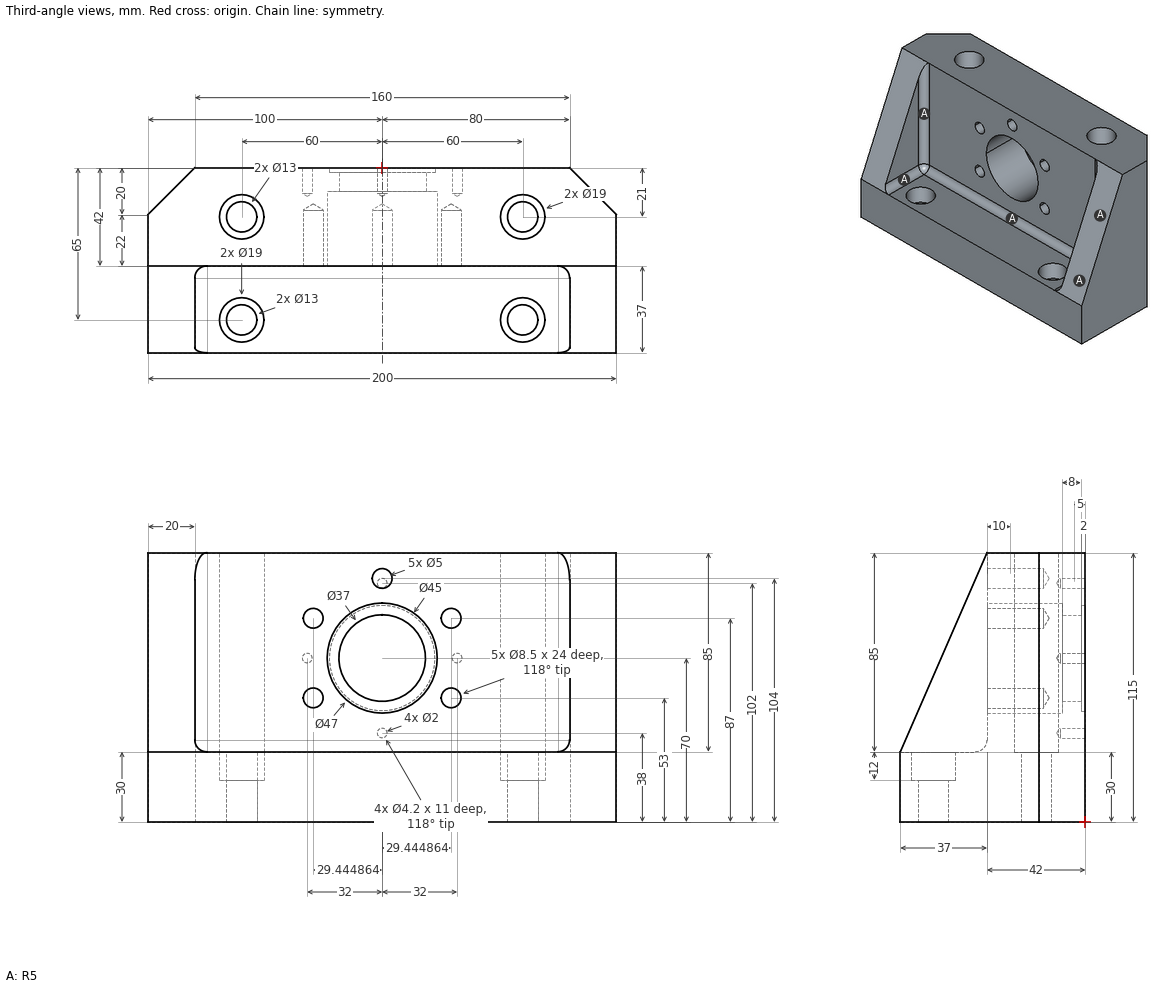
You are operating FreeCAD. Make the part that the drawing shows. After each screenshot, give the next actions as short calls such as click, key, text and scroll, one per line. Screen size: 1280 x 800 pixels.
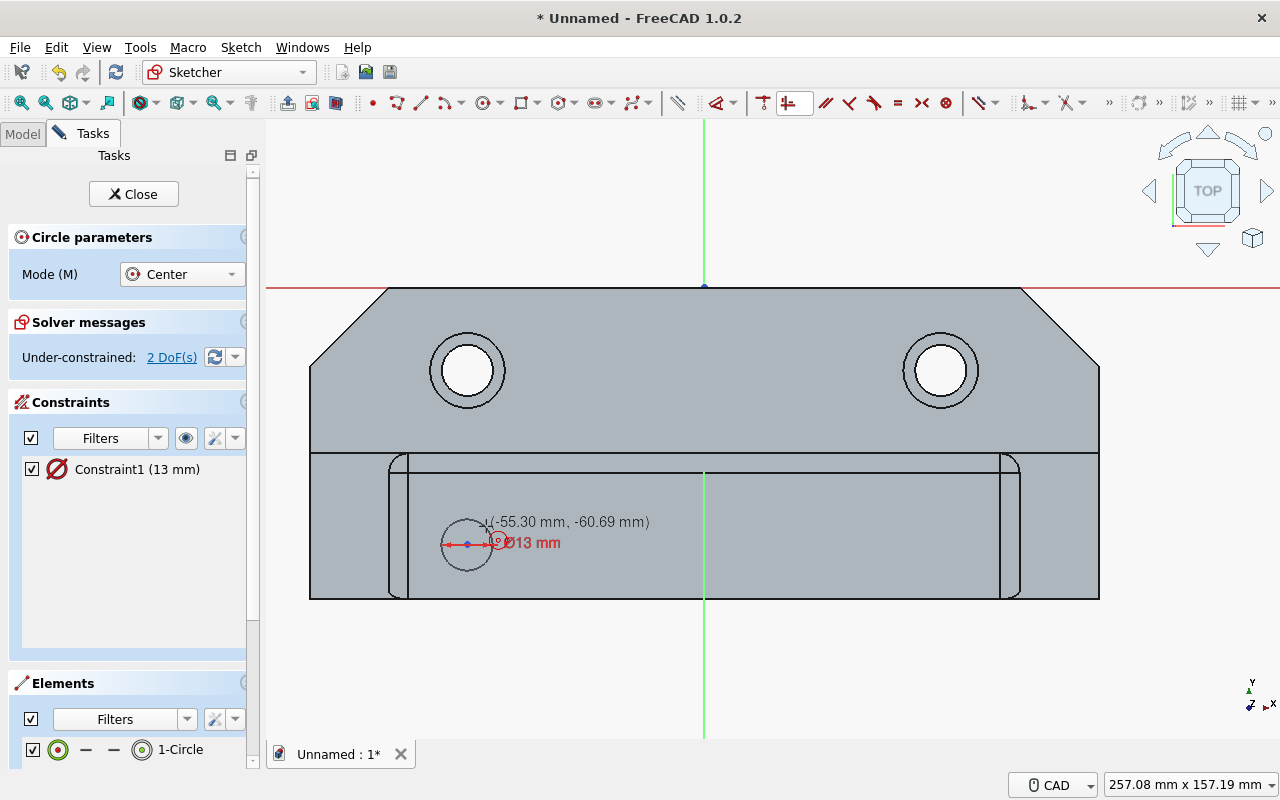
click(941, 544)
move(959, 526)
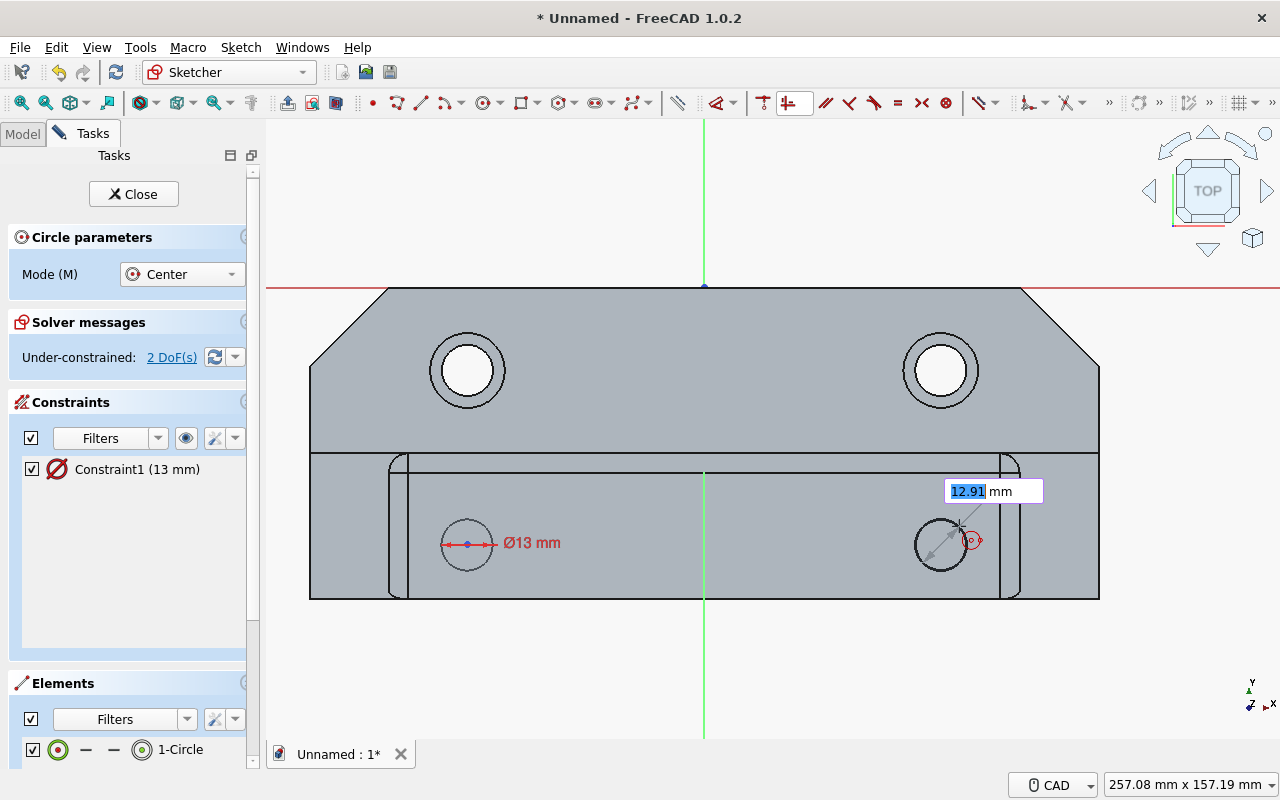
text(13)
key(Return)
key(Escape)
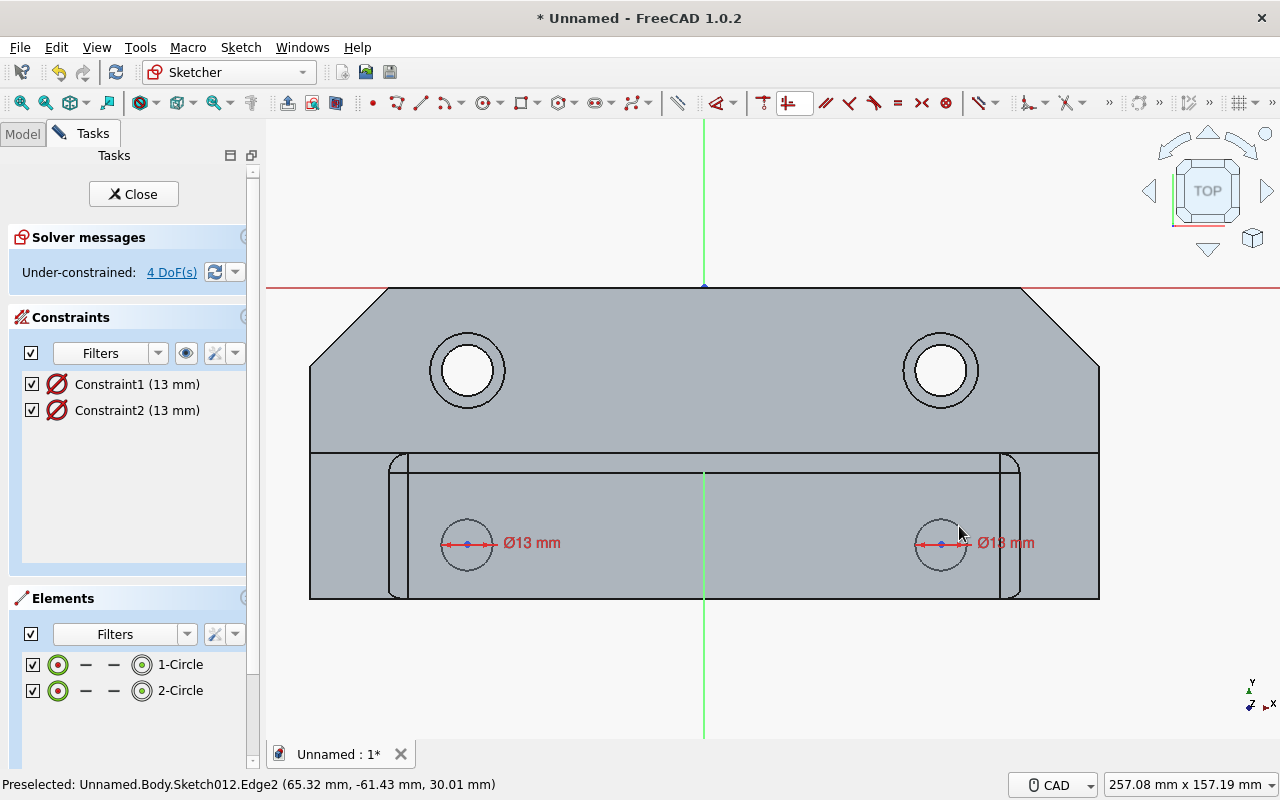
click(467, 545)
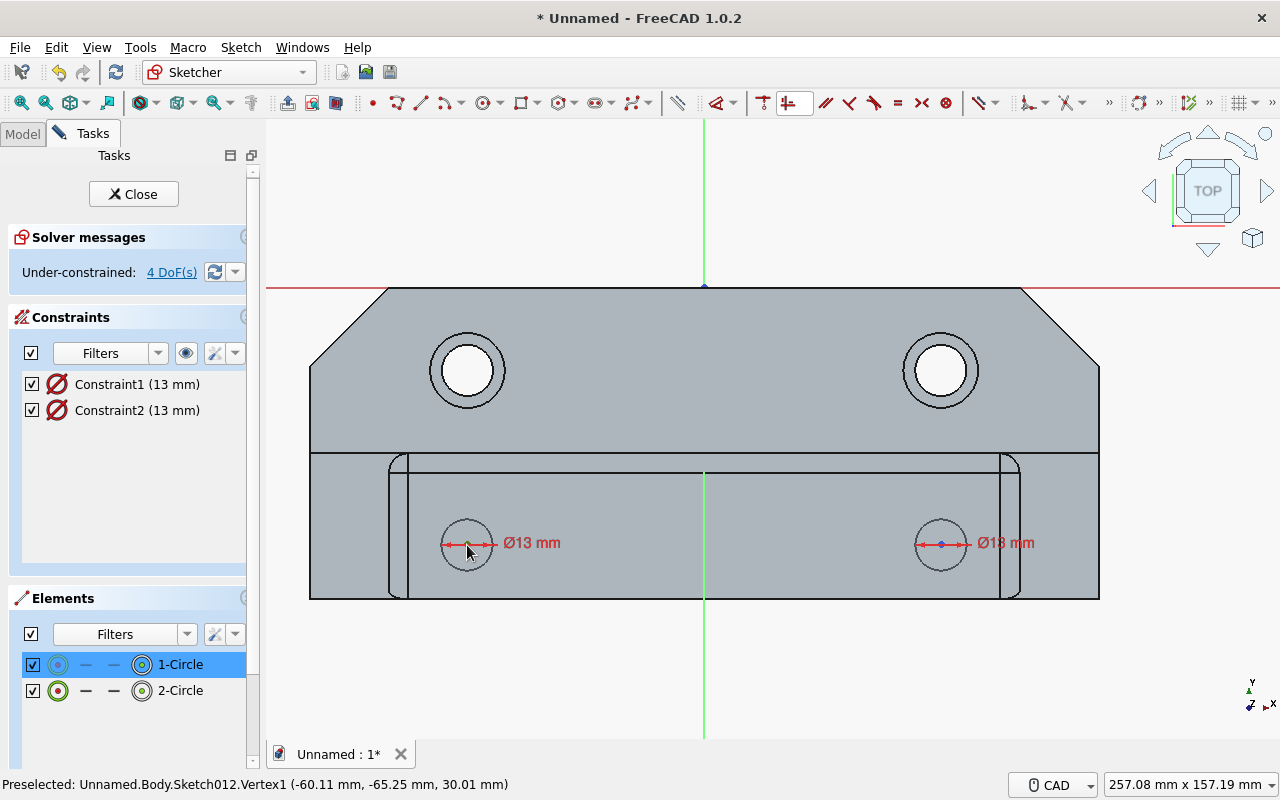
click(941, 545)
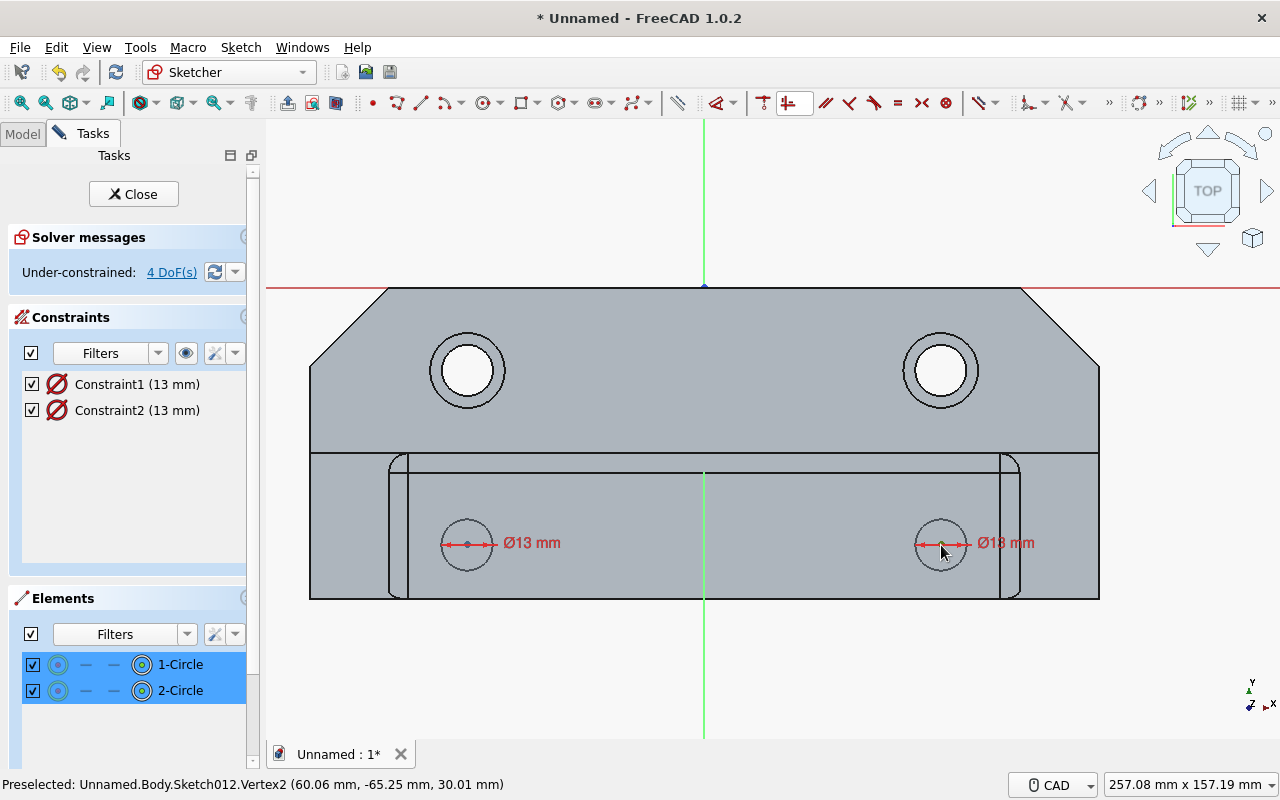
key(h)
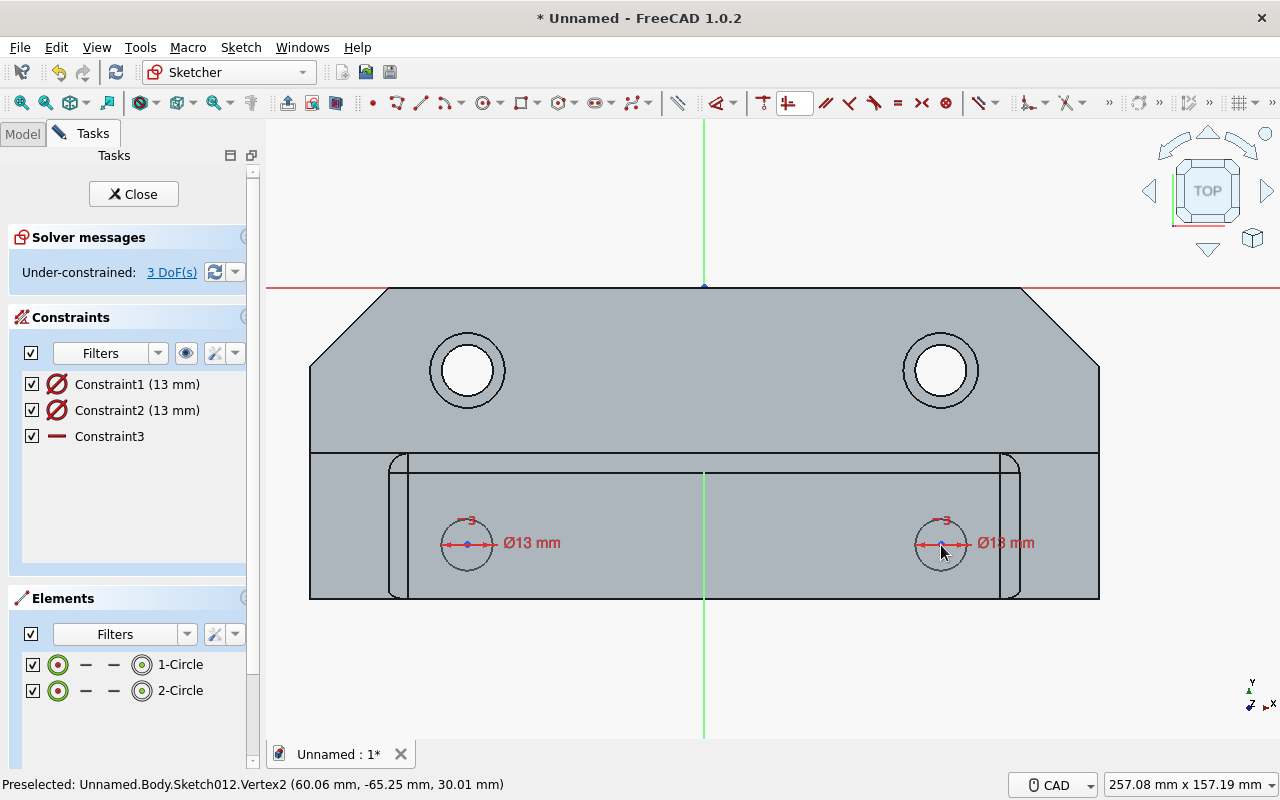
click(716, 104)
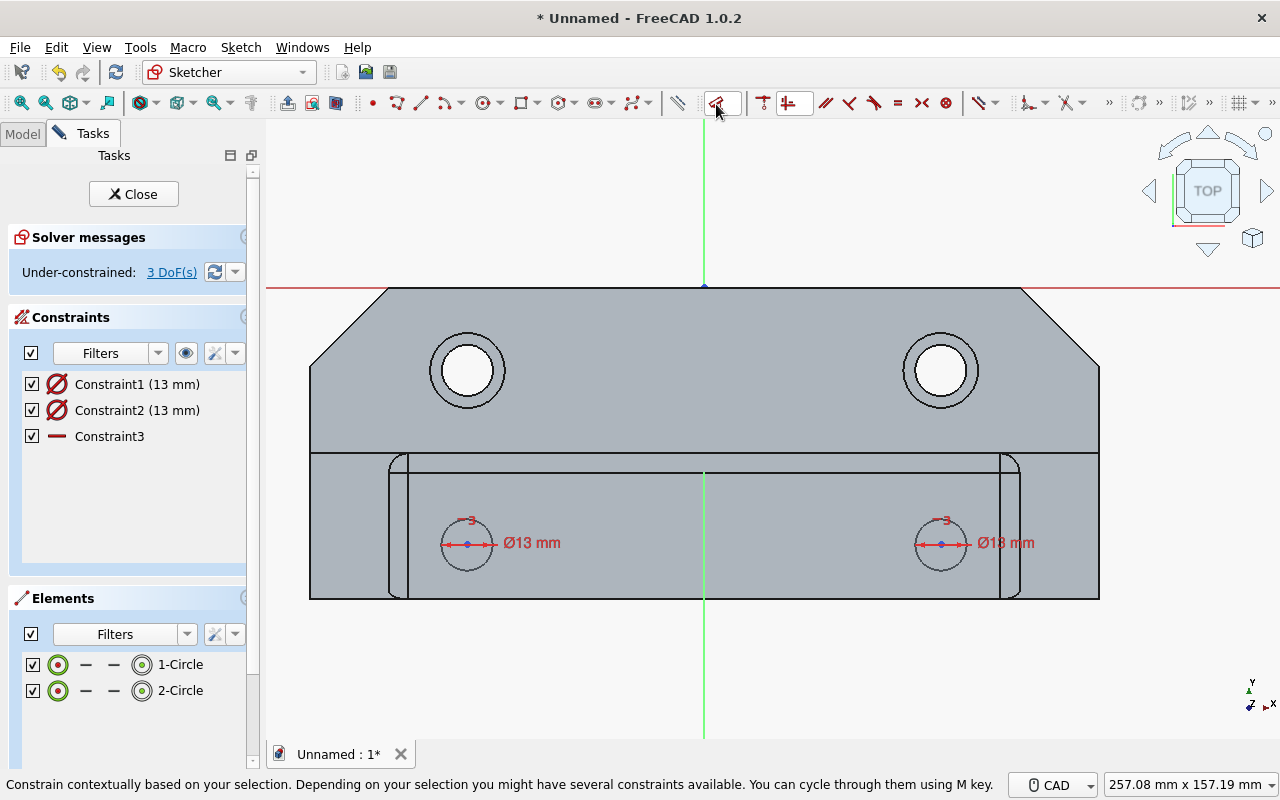
click(467, 545)
click(586, 254)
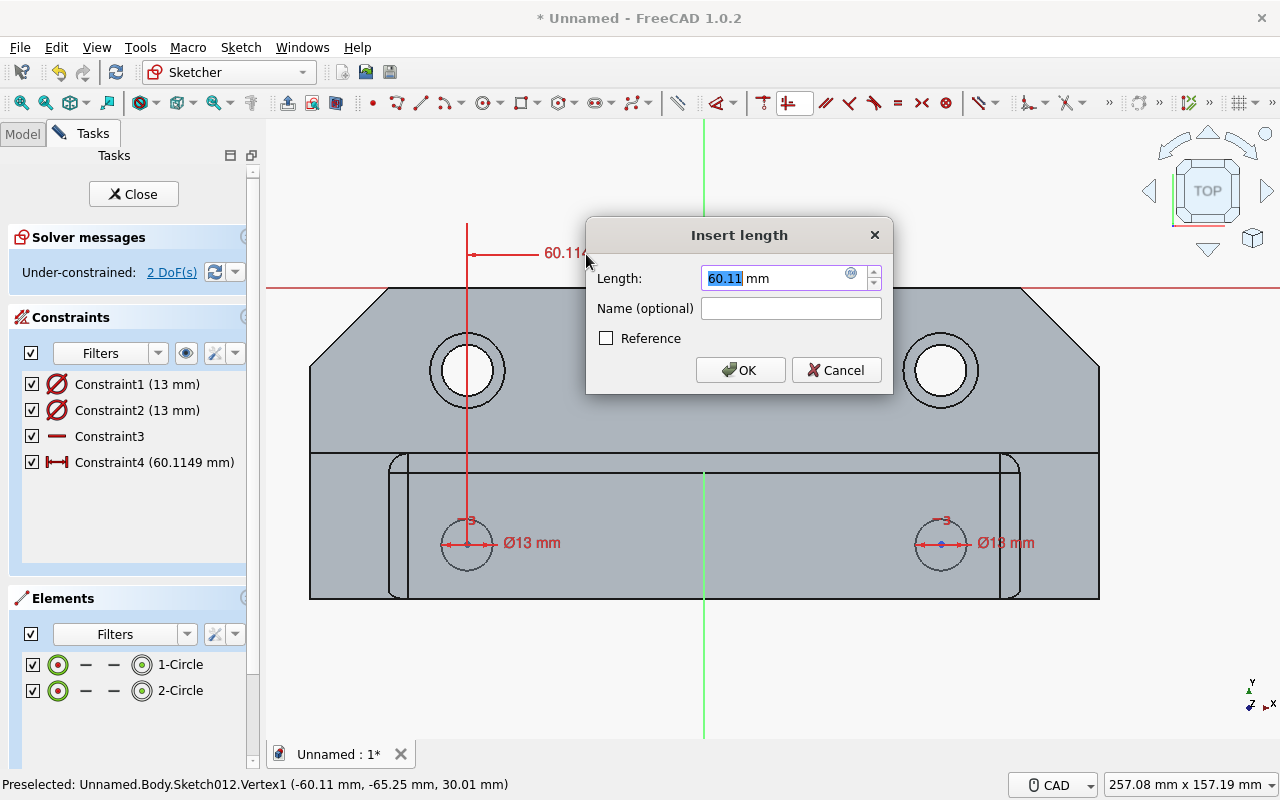
text(60)
key(Return)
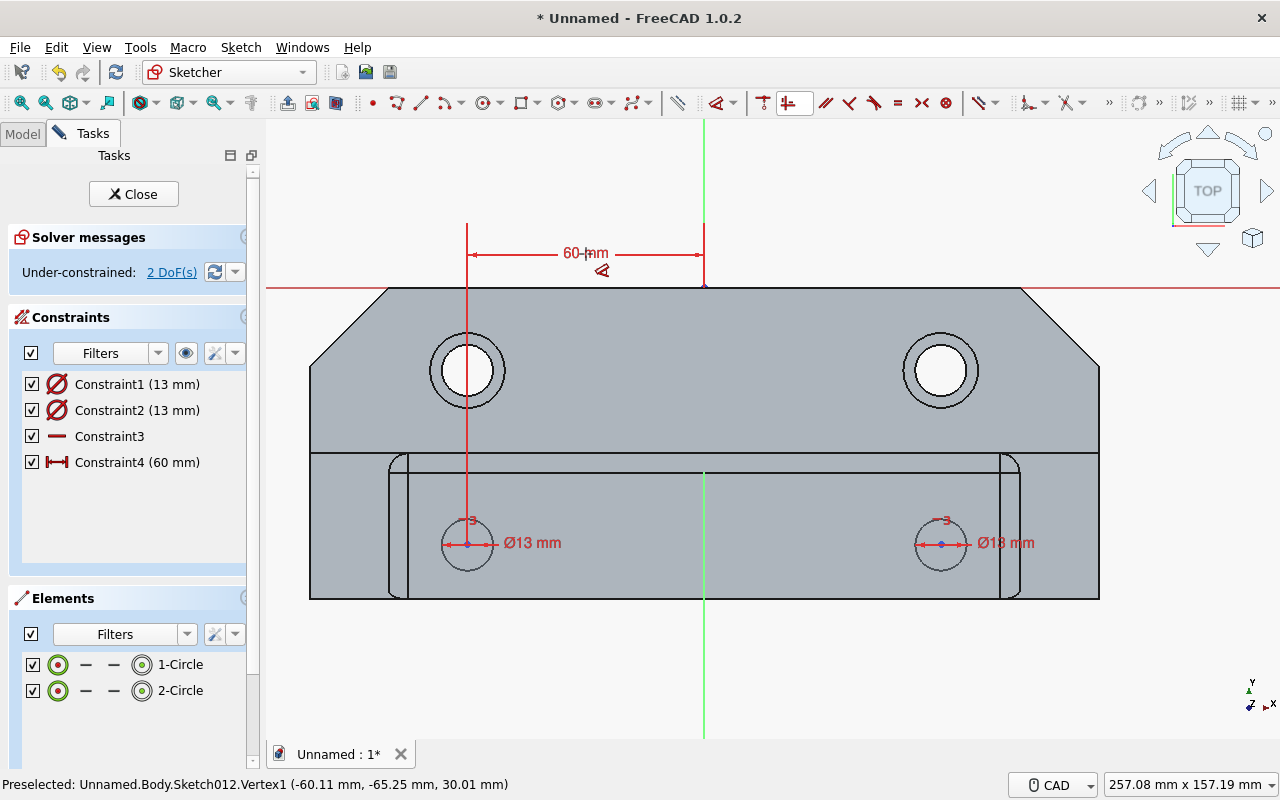
click(467, 545)
click(433, 416)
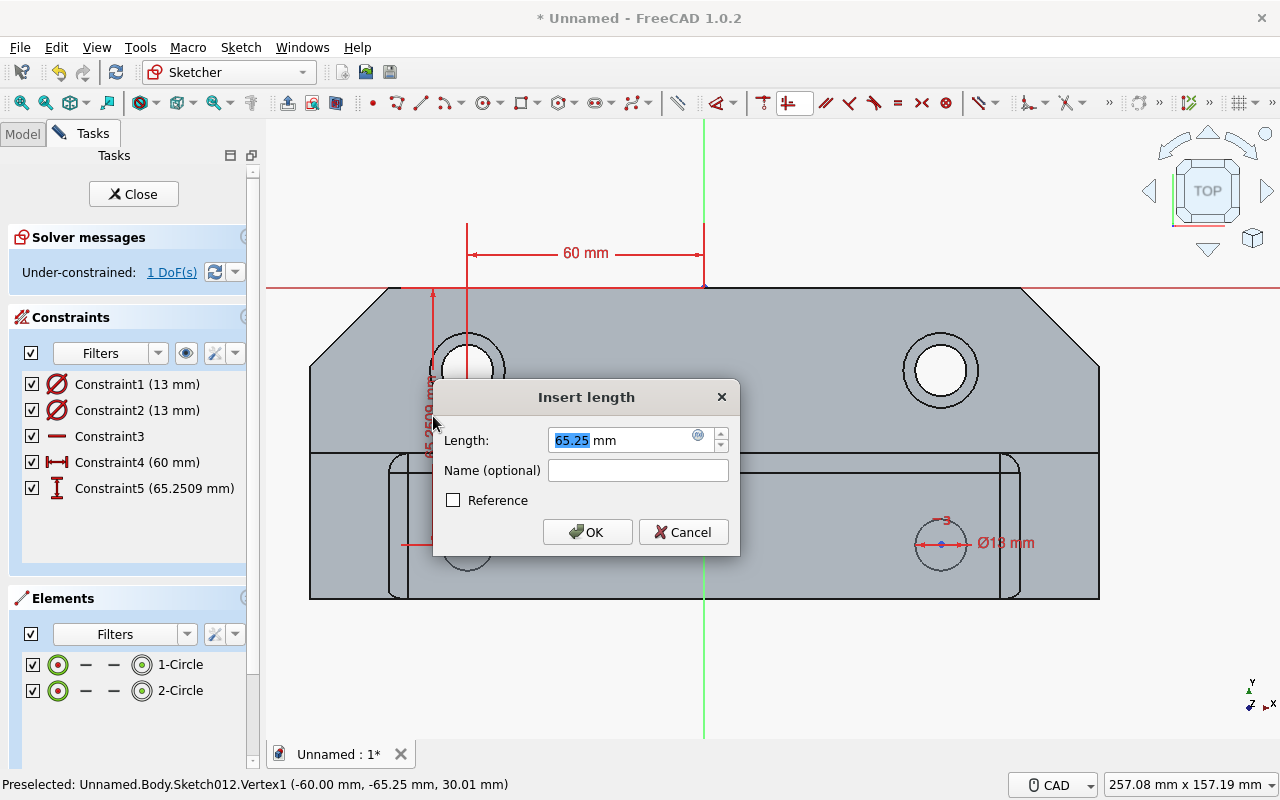
text(65)
key(Return)